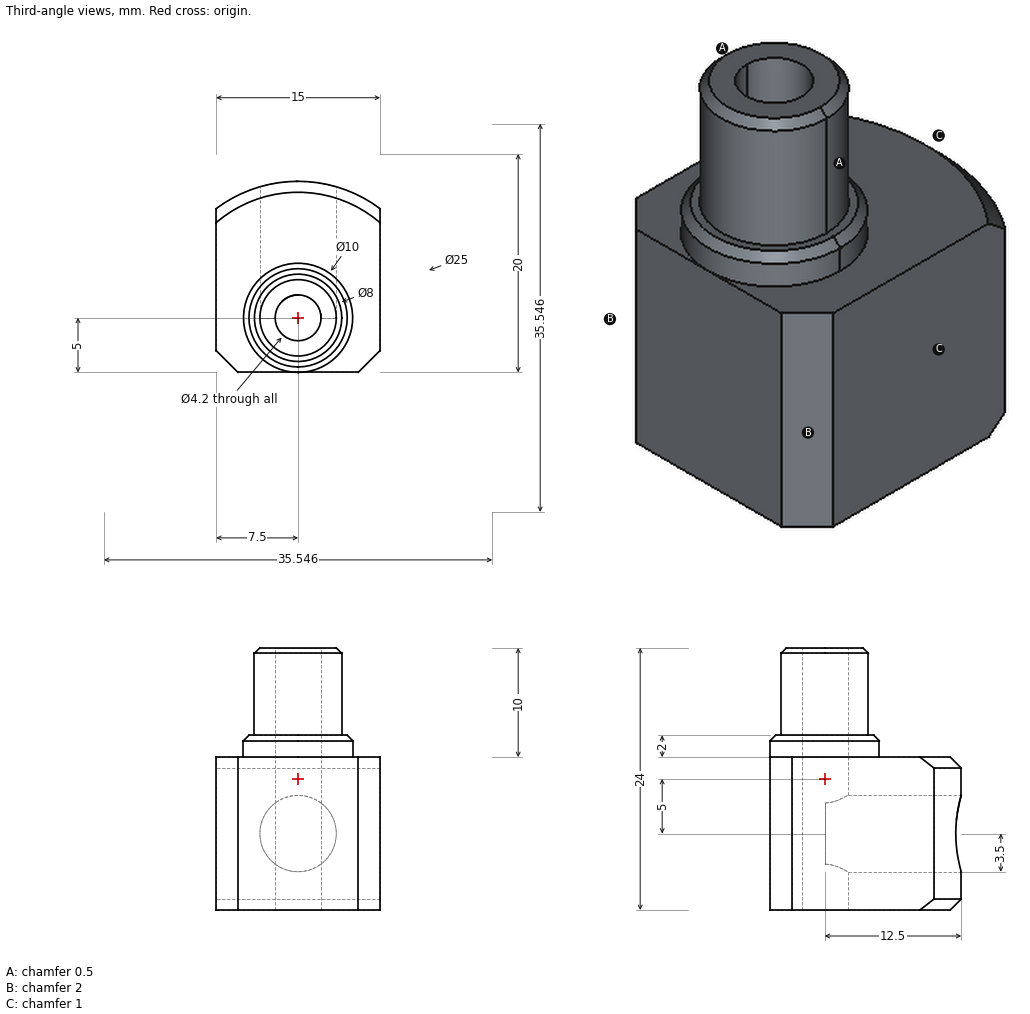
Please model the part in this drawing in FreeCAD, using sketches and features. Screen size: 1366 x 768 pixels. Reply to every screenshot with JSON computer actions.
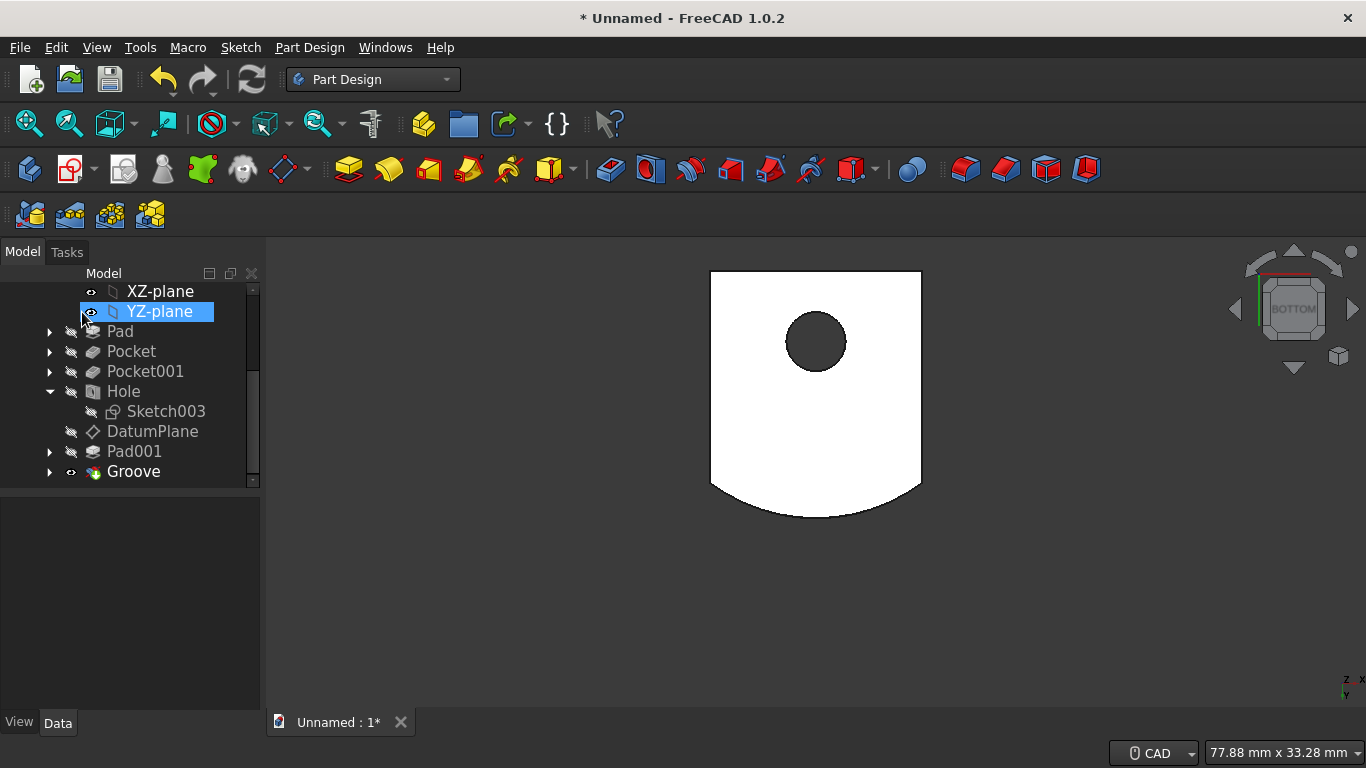
{"action": "key", "text": "0"}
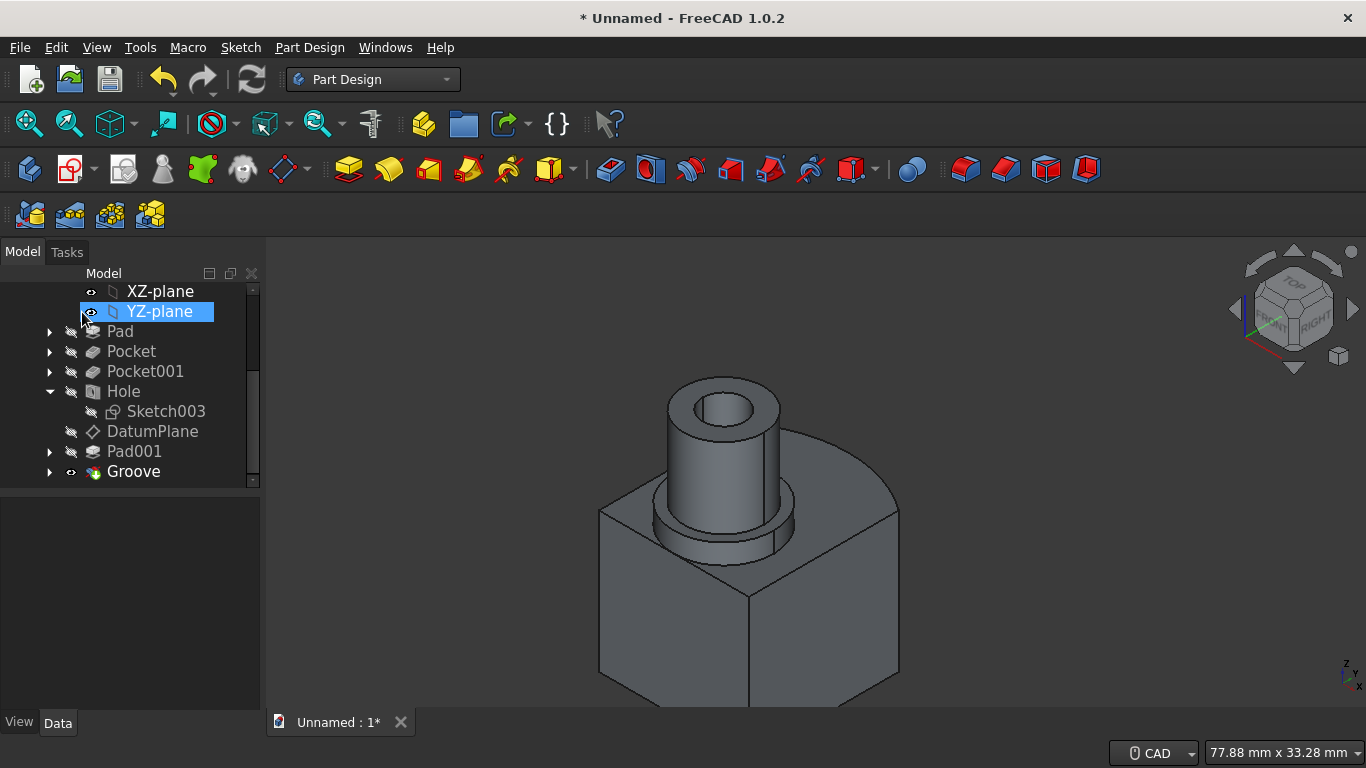
{"action": "left_click", "coordinate": [30, 124]}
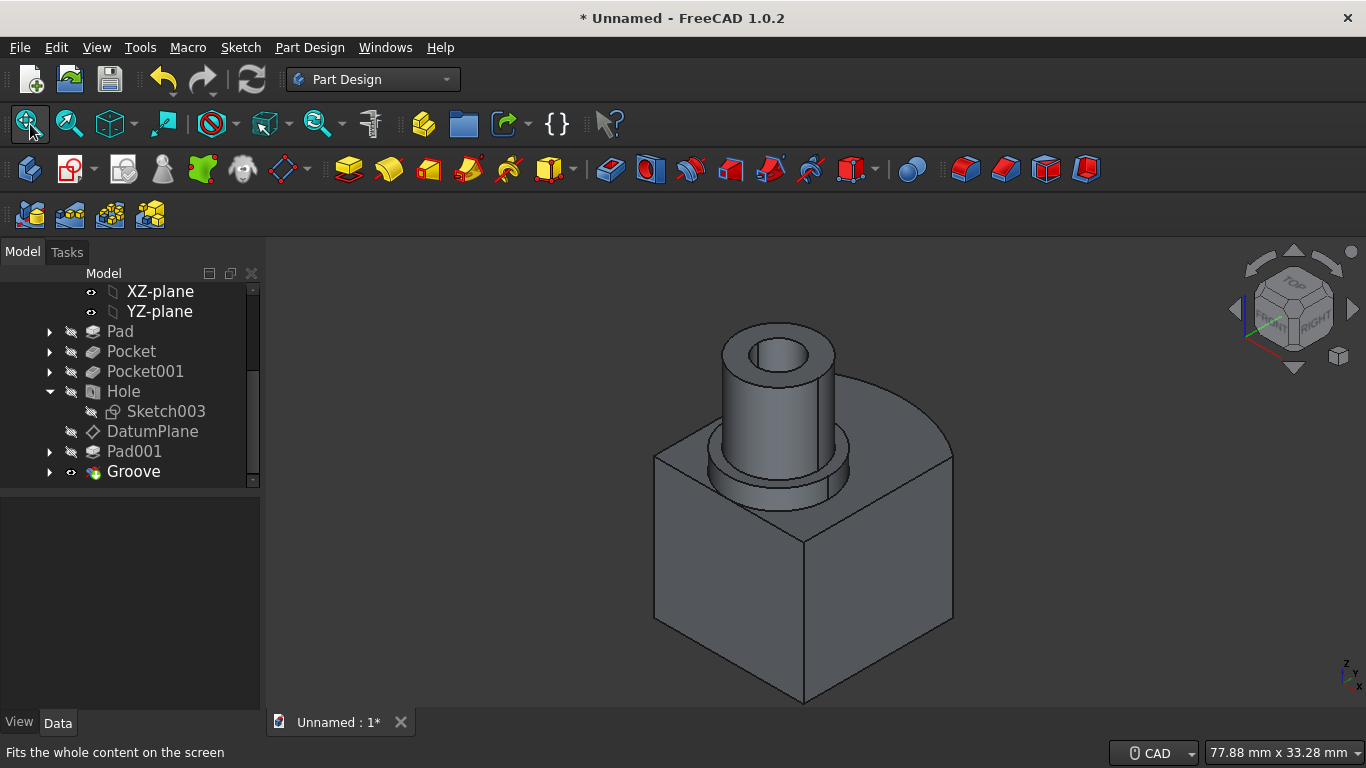
{"action": "left_click", "coordinate": [723, 349]}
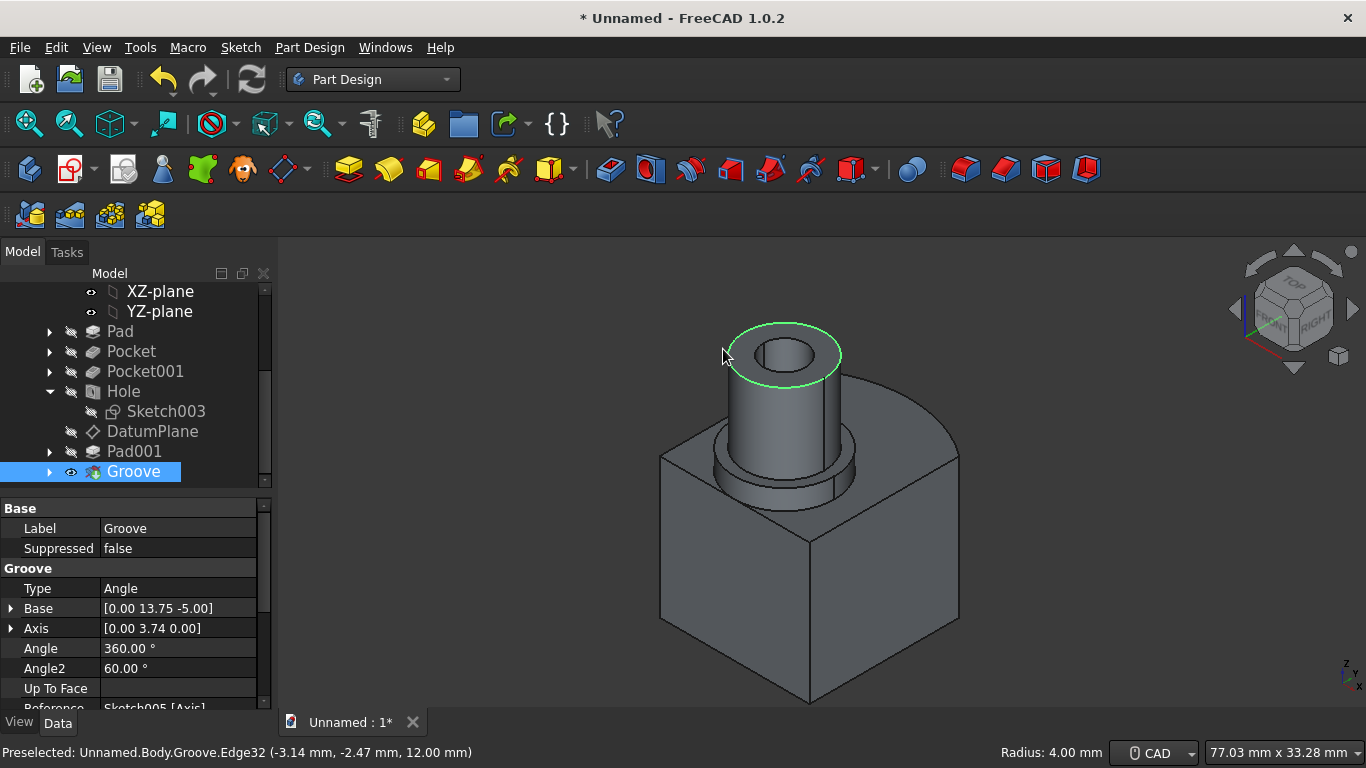
{"action": "left_click", "coordinate": [722, 465], "text": "ctrl"}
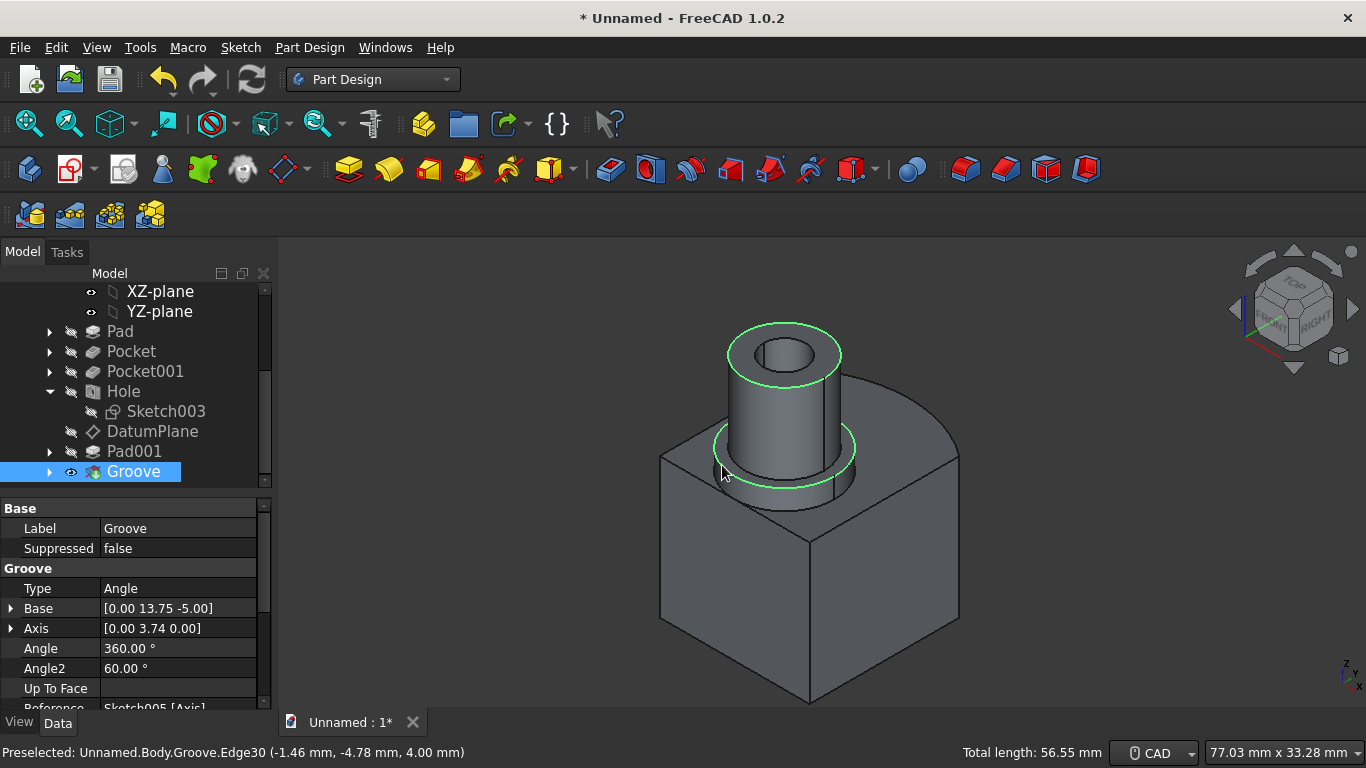
{"action": "left_click", "coordinate": [1006, 170]}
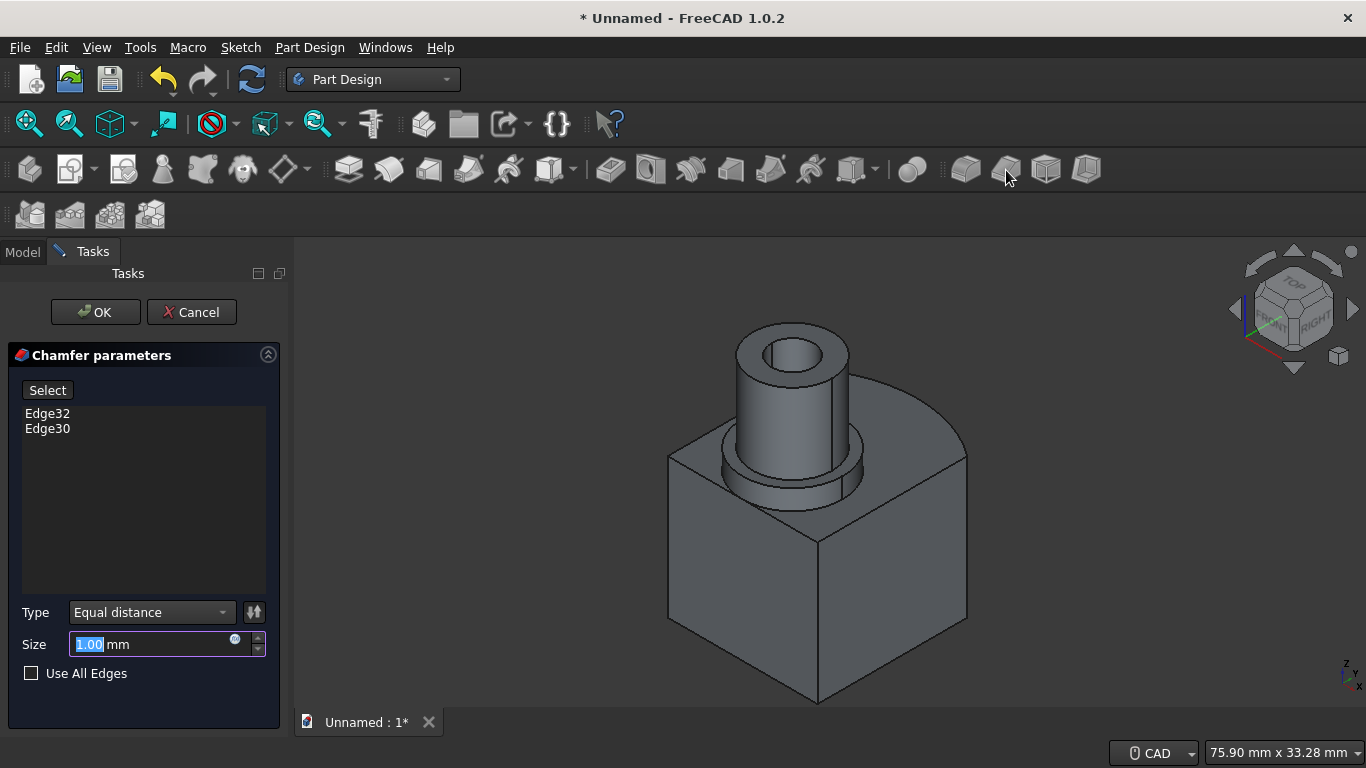
{"action": "type", "text": "0.5"}
{"action": "key", "text": "Tab"}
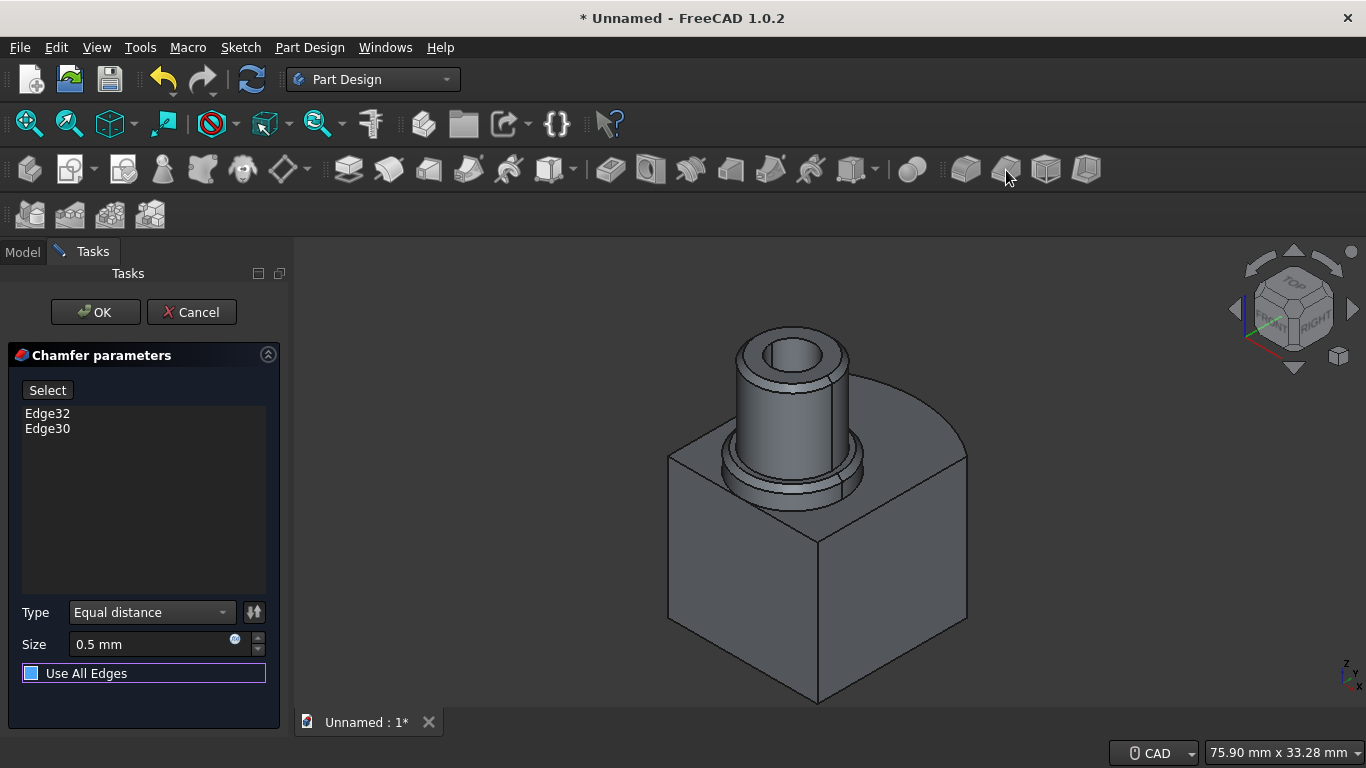
{"action": "left_click", "coordinate": [96, 312]}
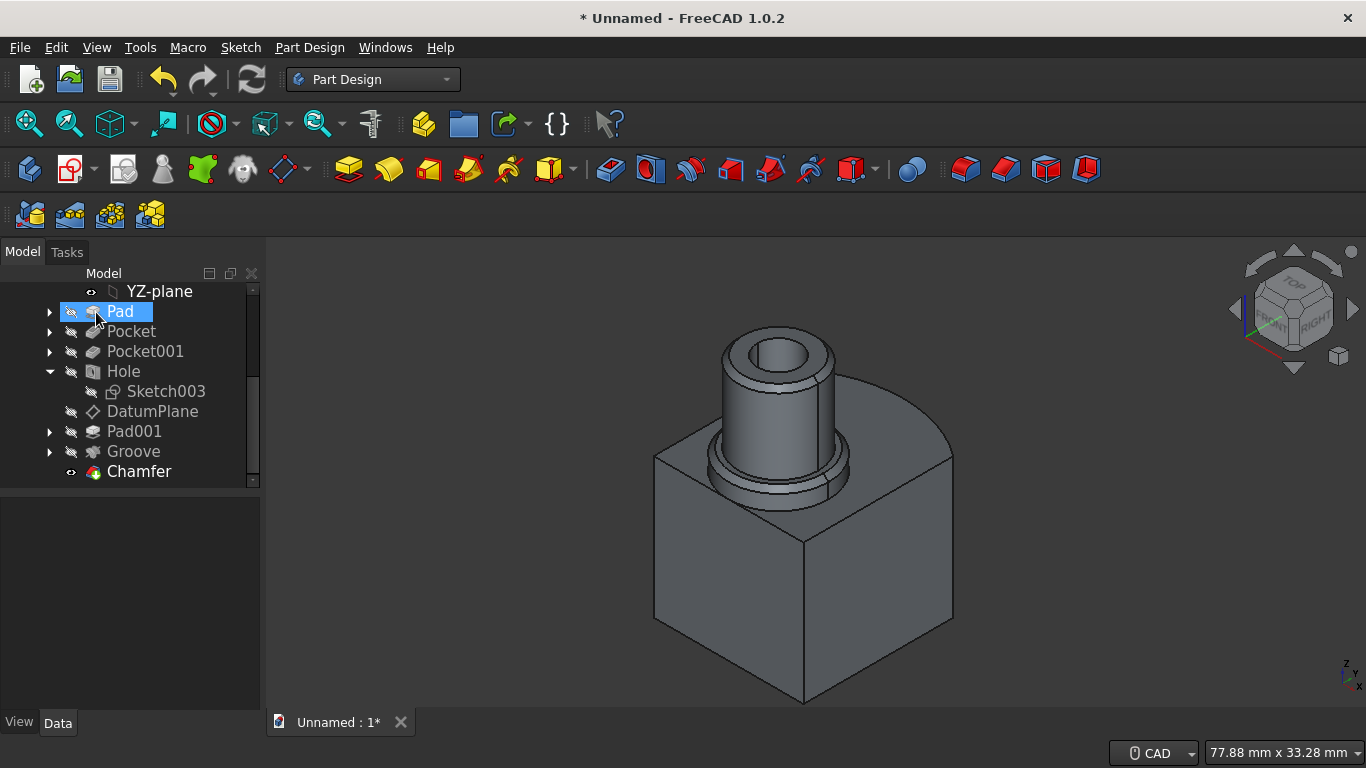
{"action": "left_click", "coordinate": [804, 622]}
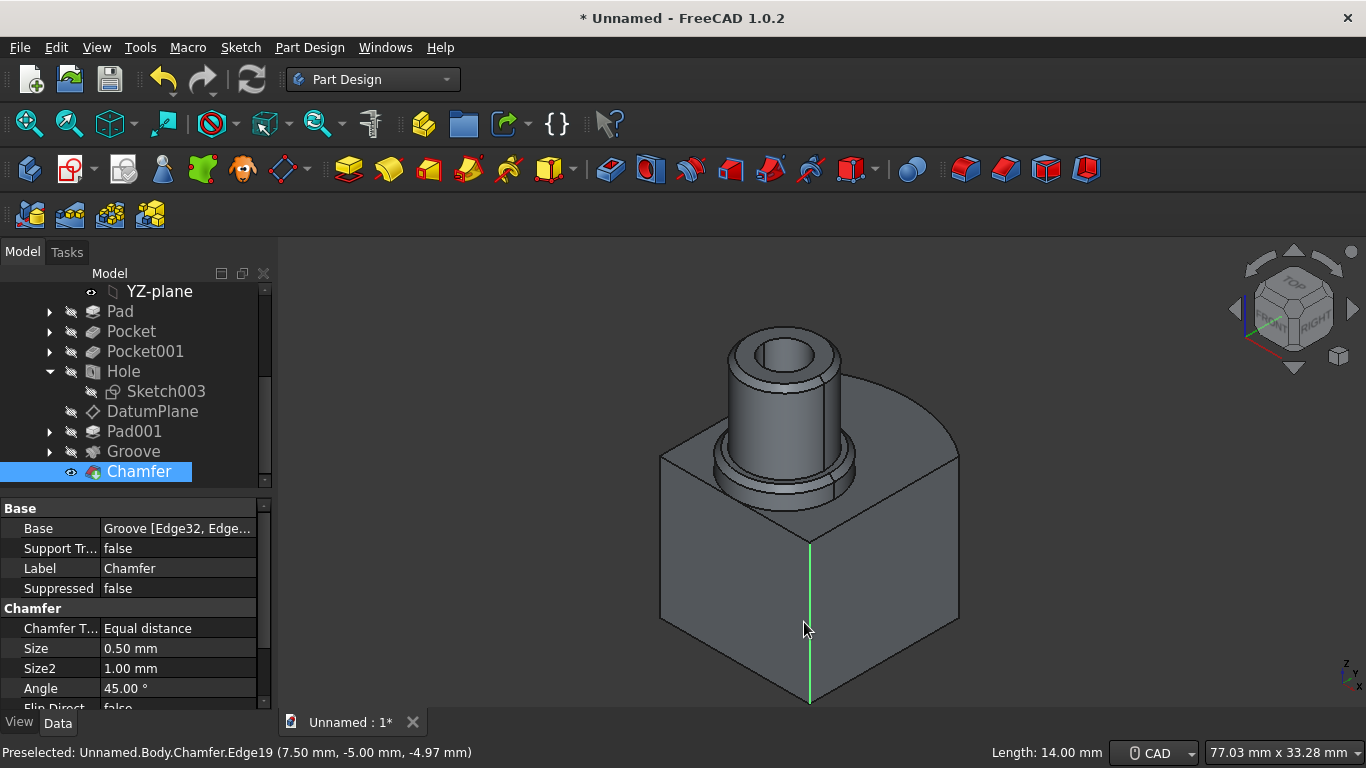
{"action": "key", "text": "2"}